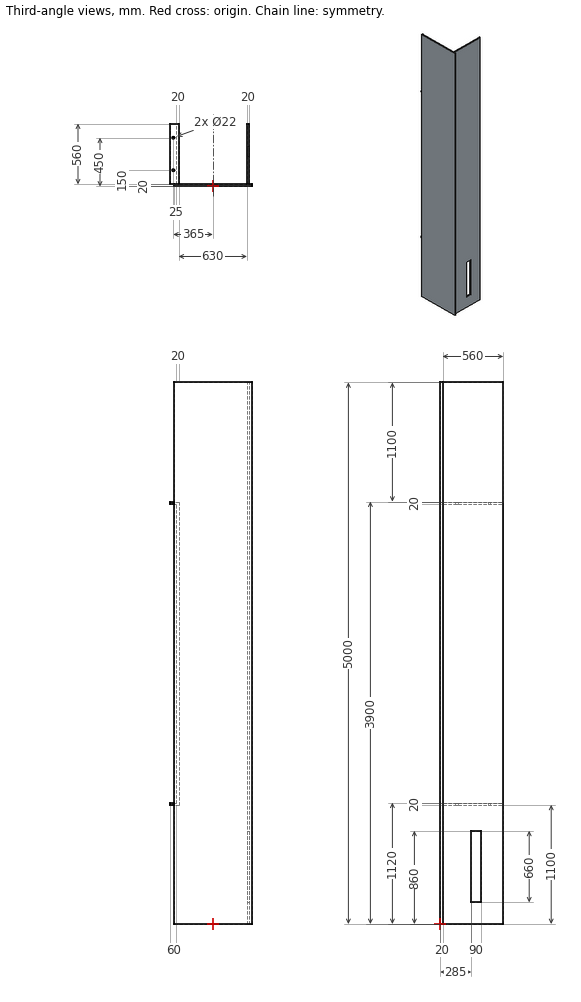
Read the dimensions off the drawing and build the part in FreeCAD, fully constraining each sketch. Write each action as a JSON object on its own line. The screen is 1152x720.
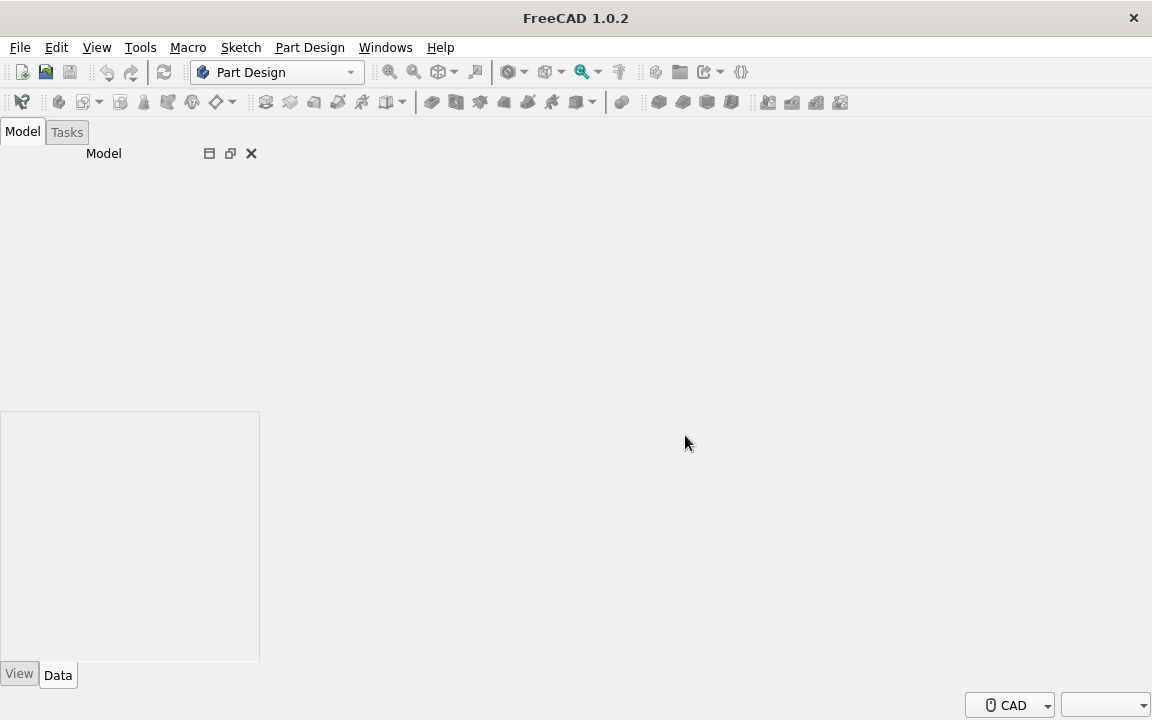
{"action": "left_click", "coordinate": [22, 72]}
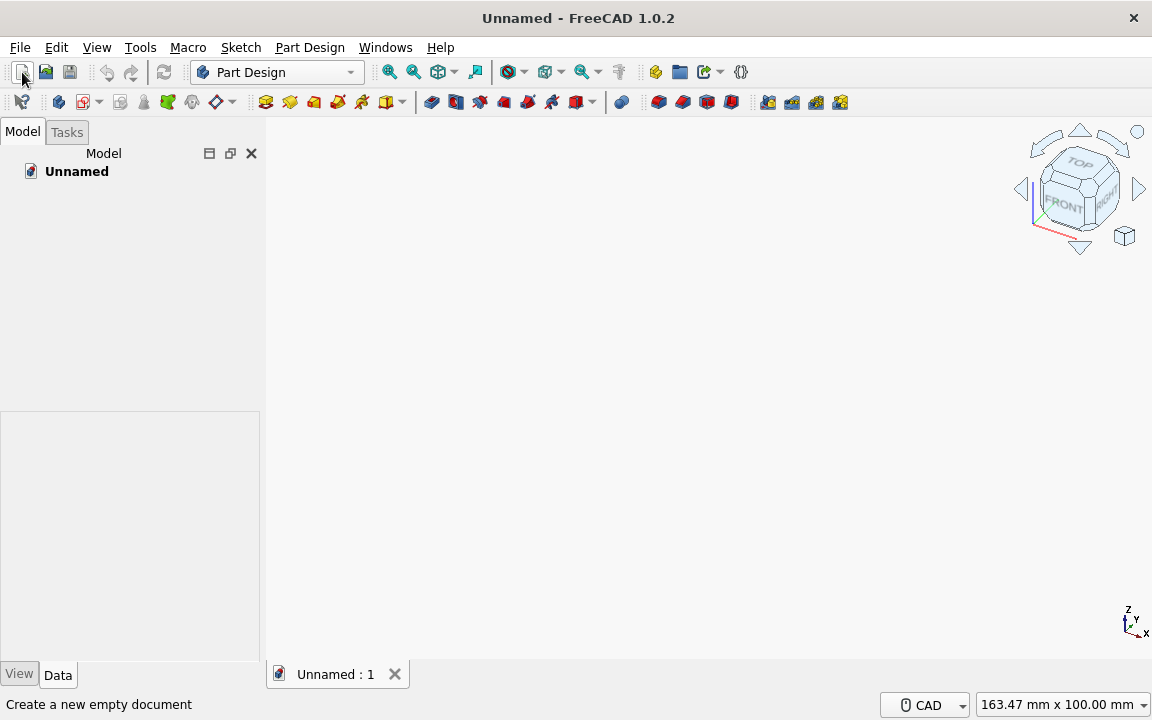
{"action": "left_click", "coordinate": [84, 102]}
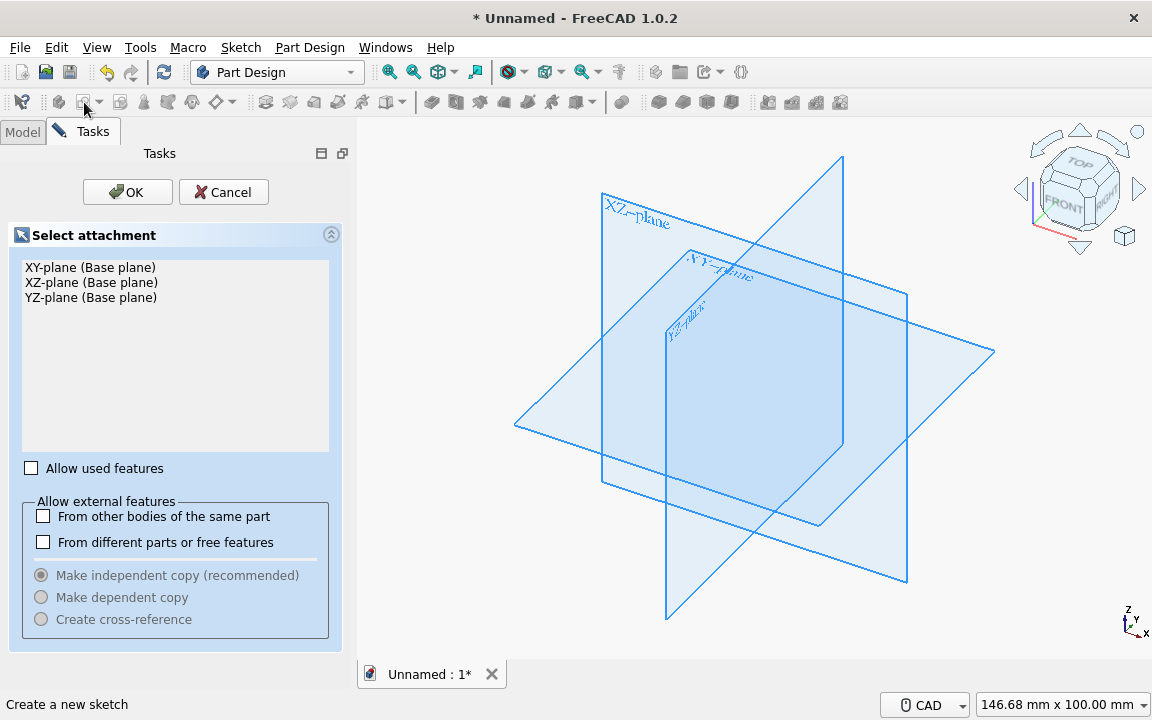
{"action": "left_click", "coordinate": [82, 268]}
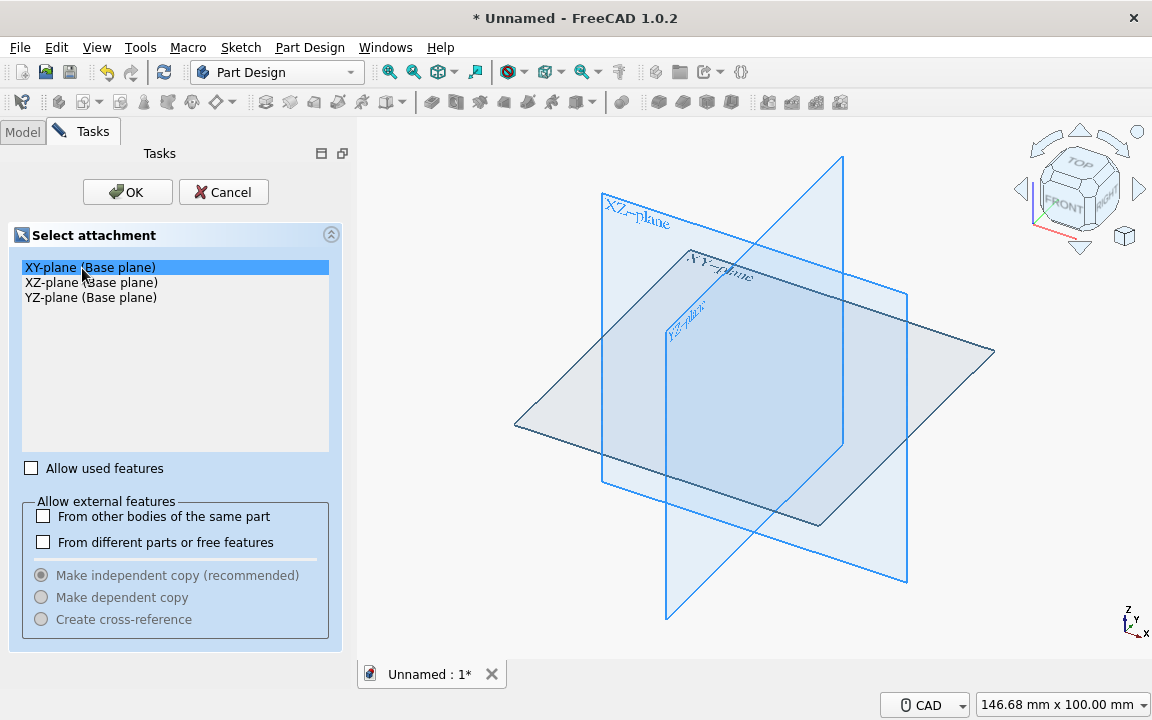
{"action": "left_click", "coordinate": [128, 192]}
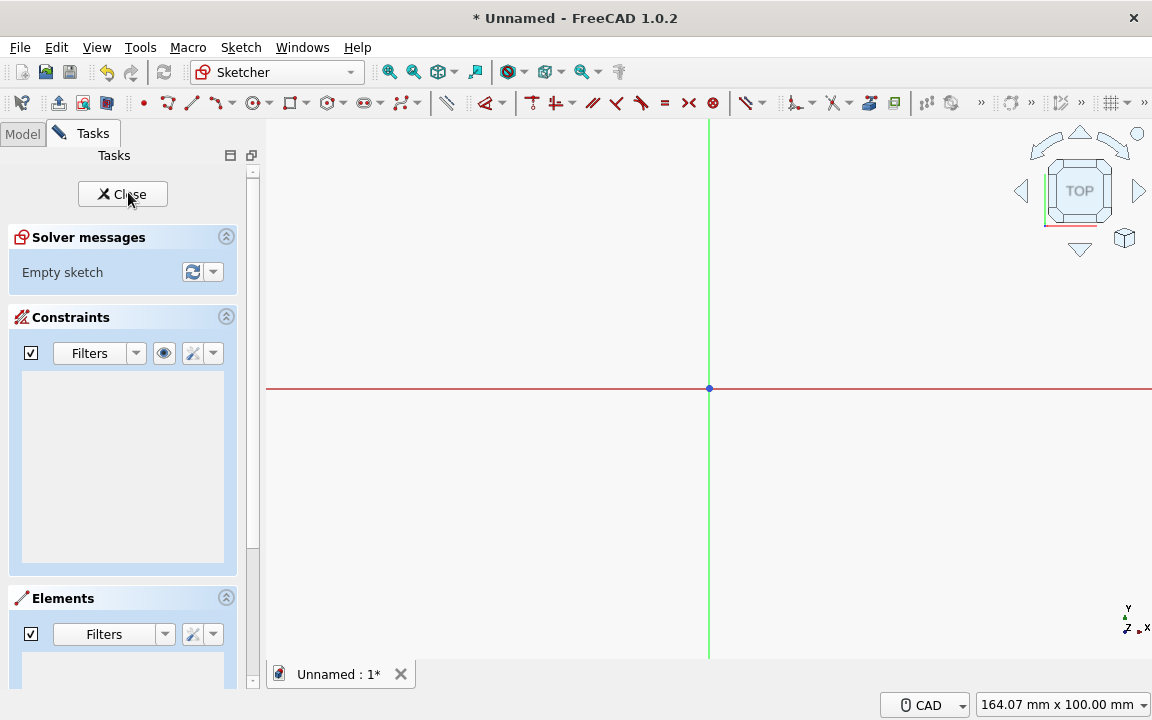
{"action": "scroll", "coordinate": [632, 584], "scroll_direction": "down", "scroll_amount": 11}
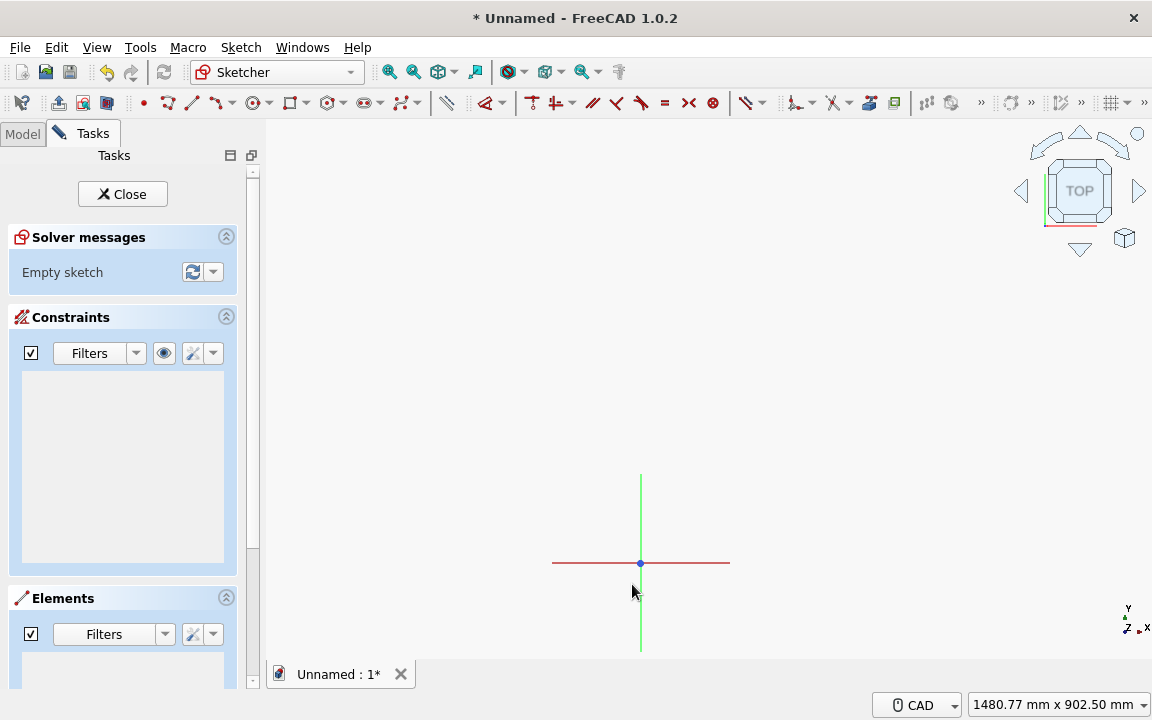
{"action": "left_click", "coordinate": [168, 104]}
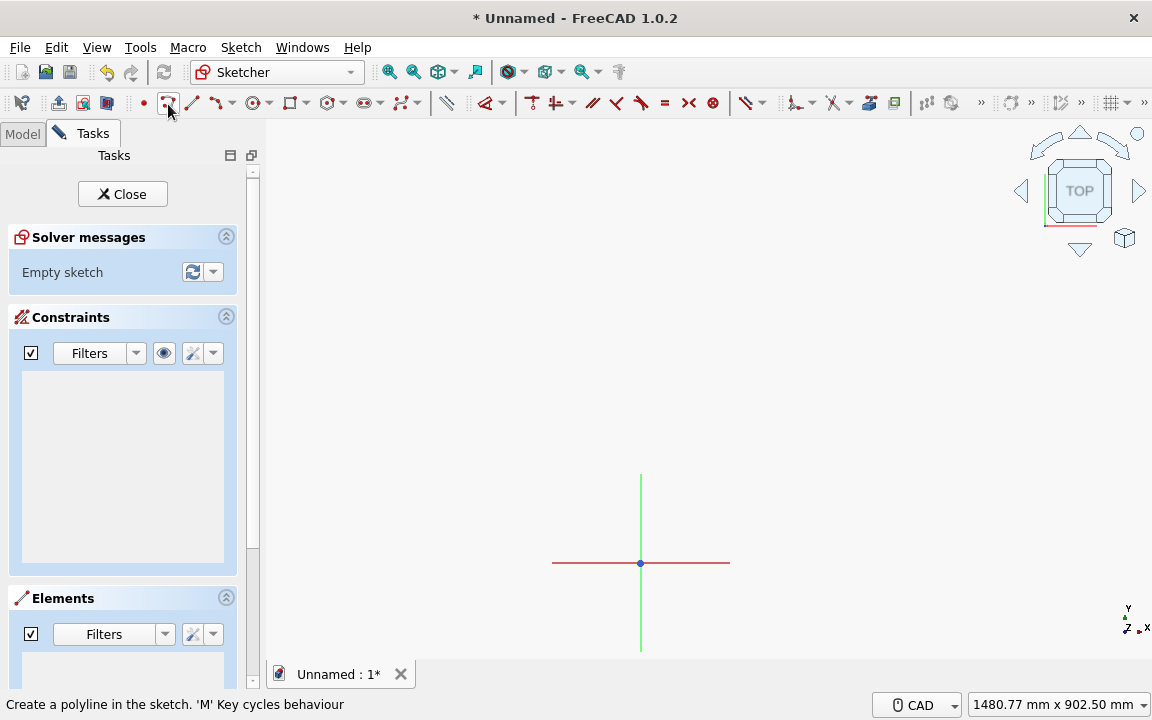
{"action": "scroll", "coordinate": [829, 551], "scroll_direction": "up", "scroll_amount": 2}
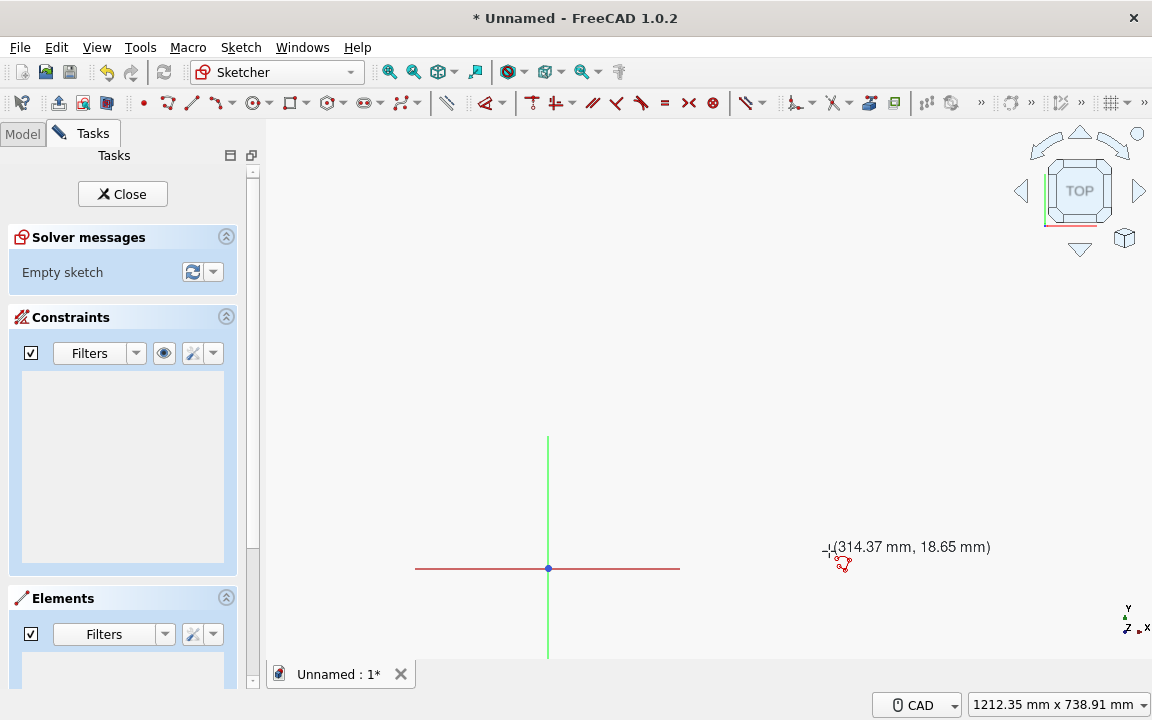
{"action": "left_click", "coordinate": [829, 551]}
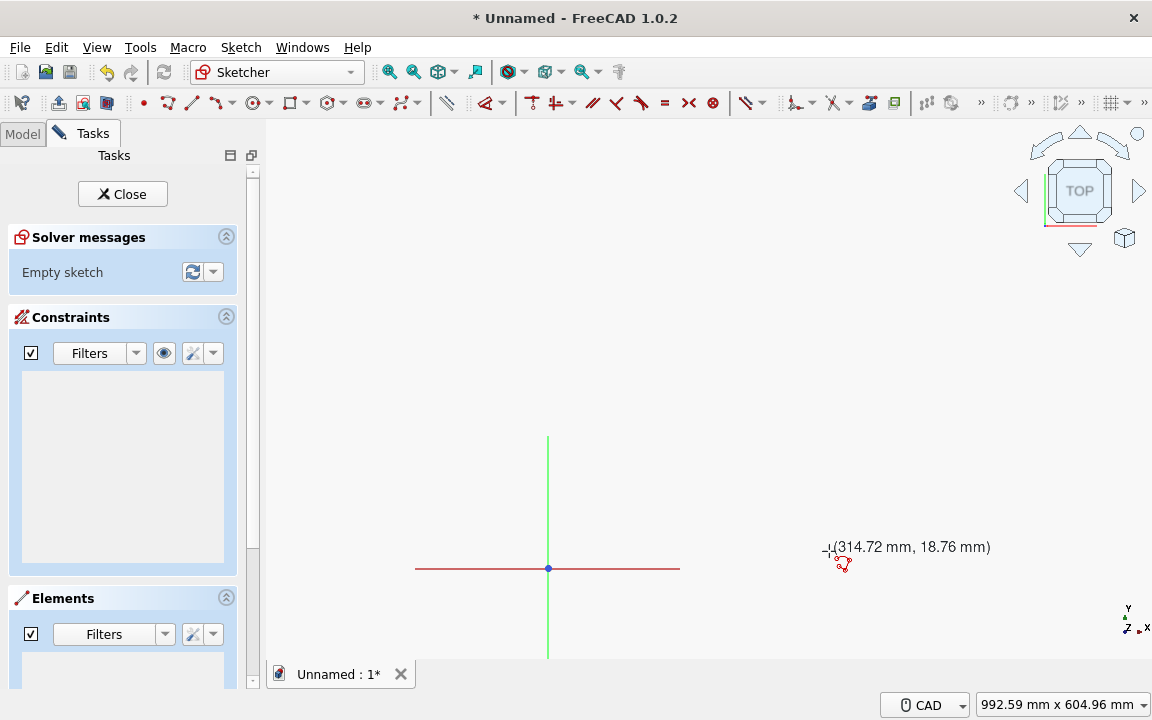
{"action": "scroll", "coordinate": [828, 550], "scroll_direction": "down", "scroll_amount": 2}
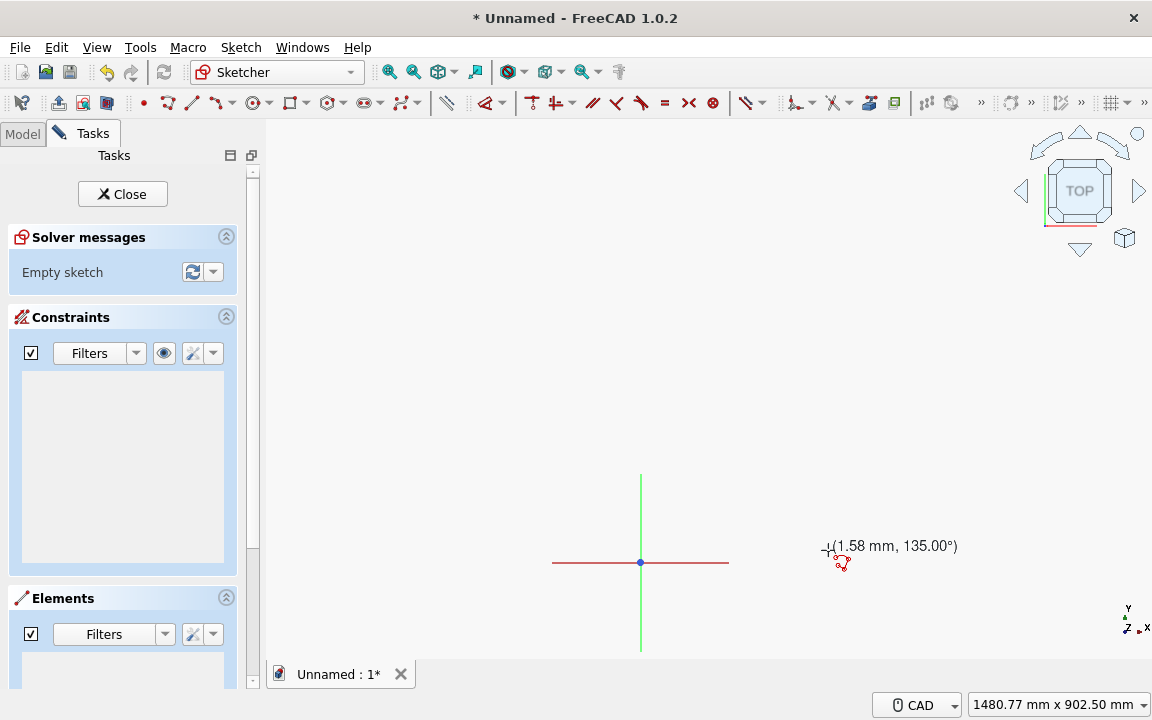
{"action": "scroll", "coordinate": [452, 551], "scroll_direction": "up", "scroll_amount": 2}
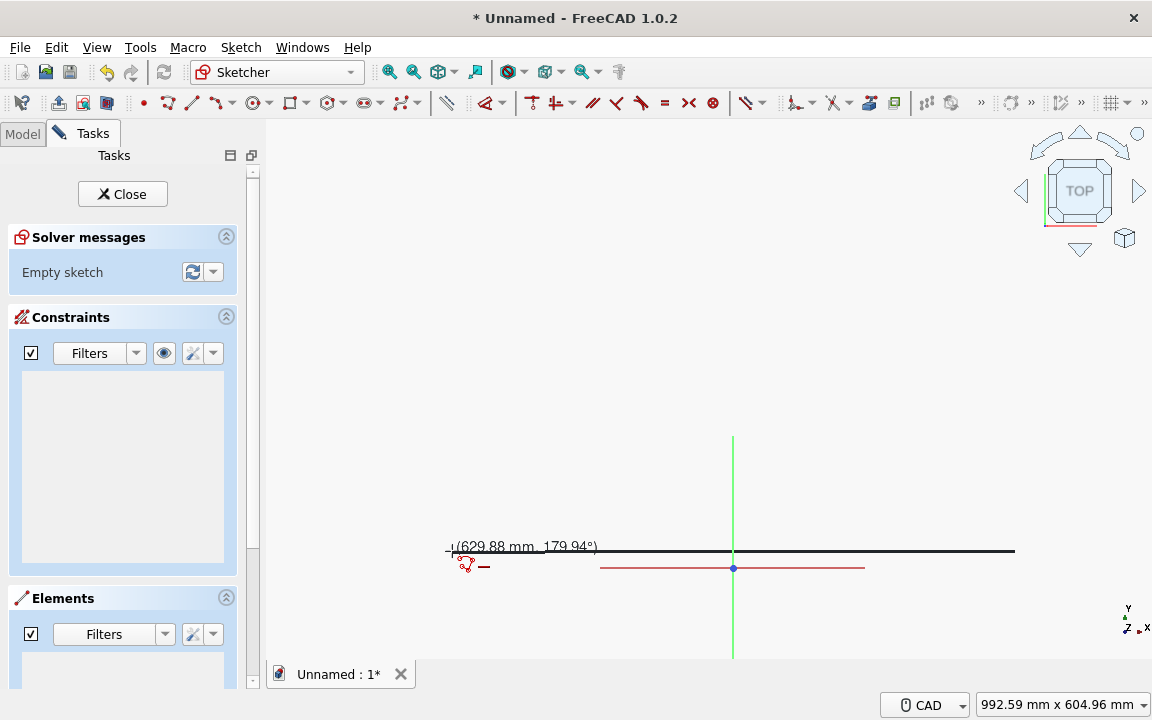
{"action": "left_click", "coordinate": [452, 551]}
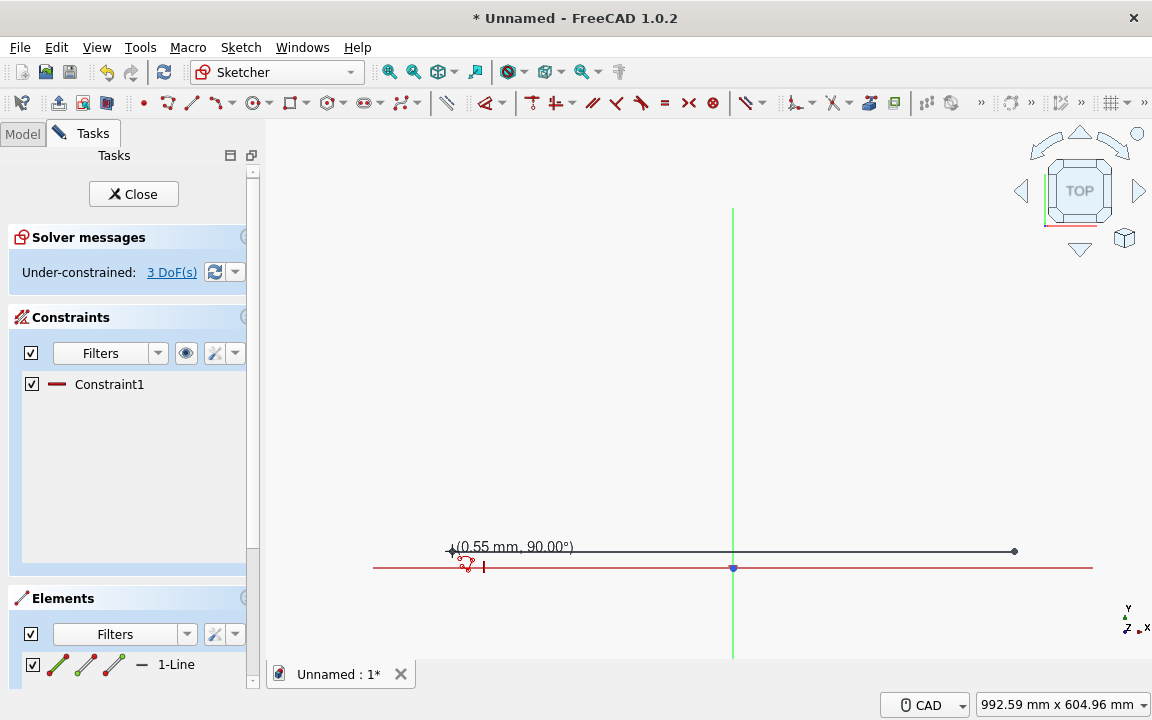
{"action": "scroll", "coordinate": [452, 551], "scroll_direction": "down", "scroll_amount": 2}